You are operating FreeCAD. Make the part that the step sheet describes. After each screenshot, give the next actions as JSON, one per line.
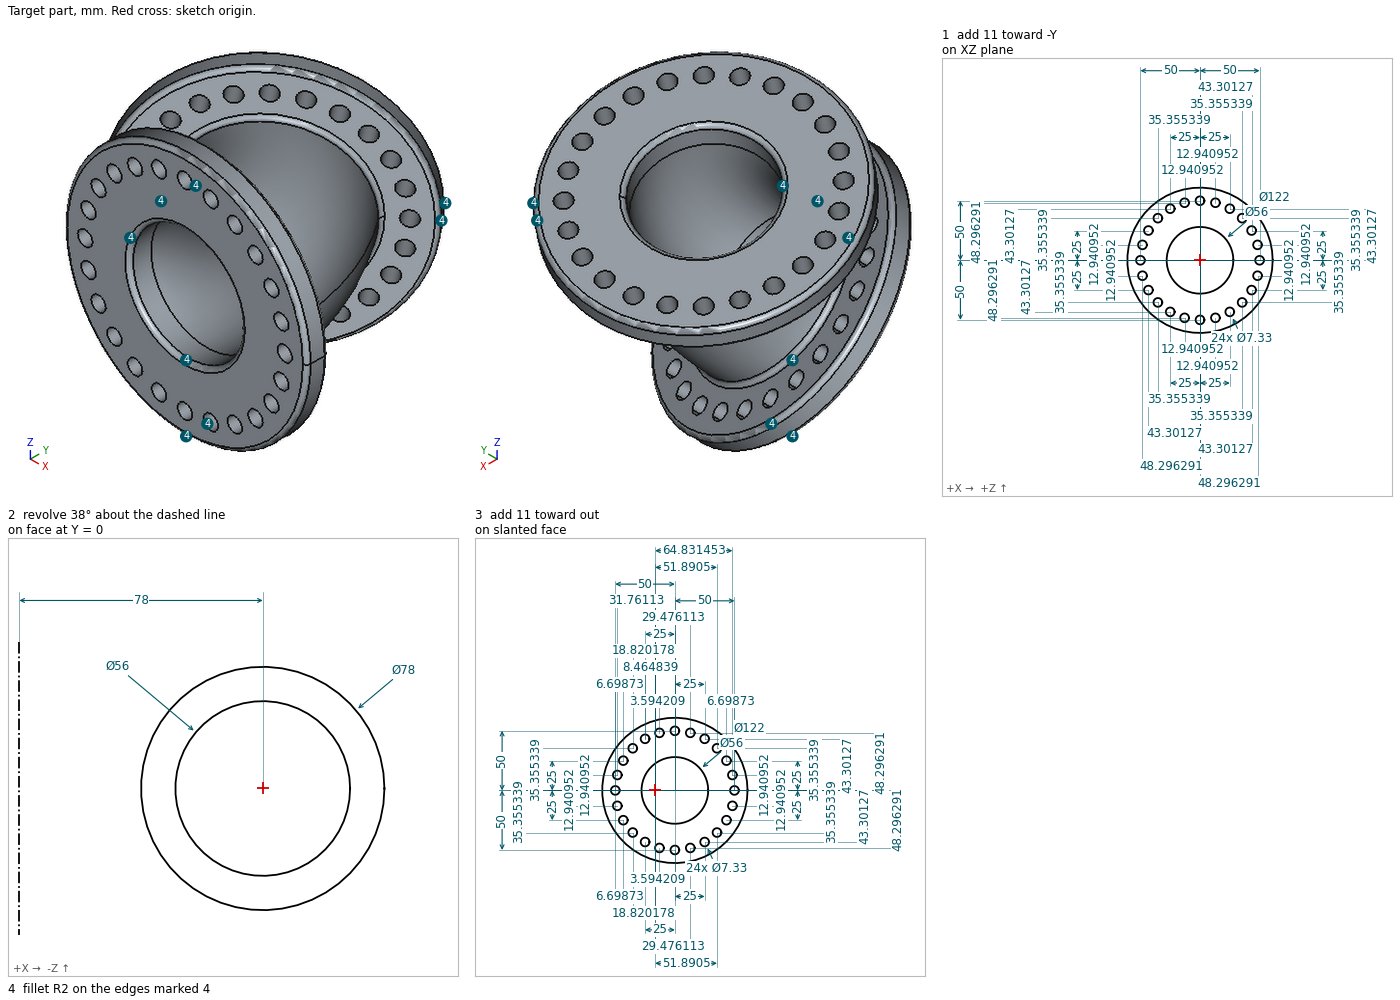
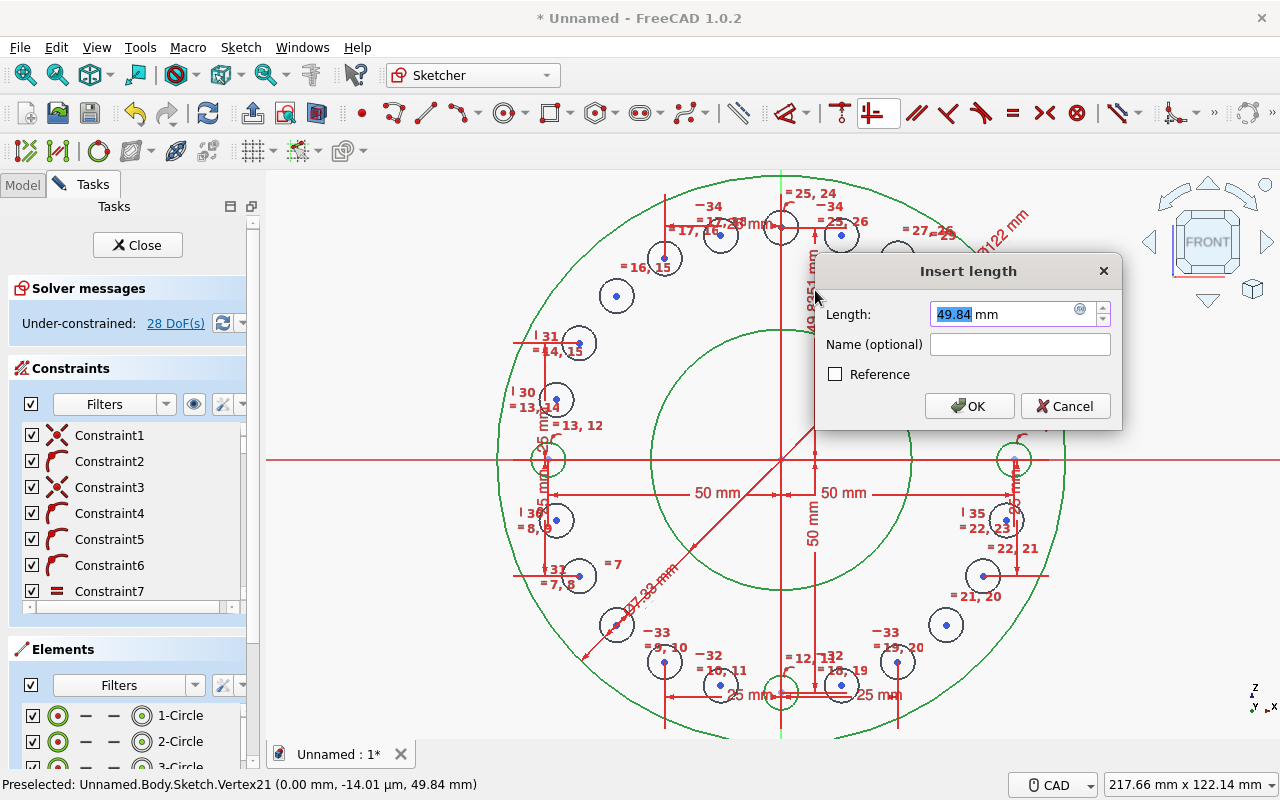
{"action": "type", "text": "50"}
{"action": "key", "text": "Return"}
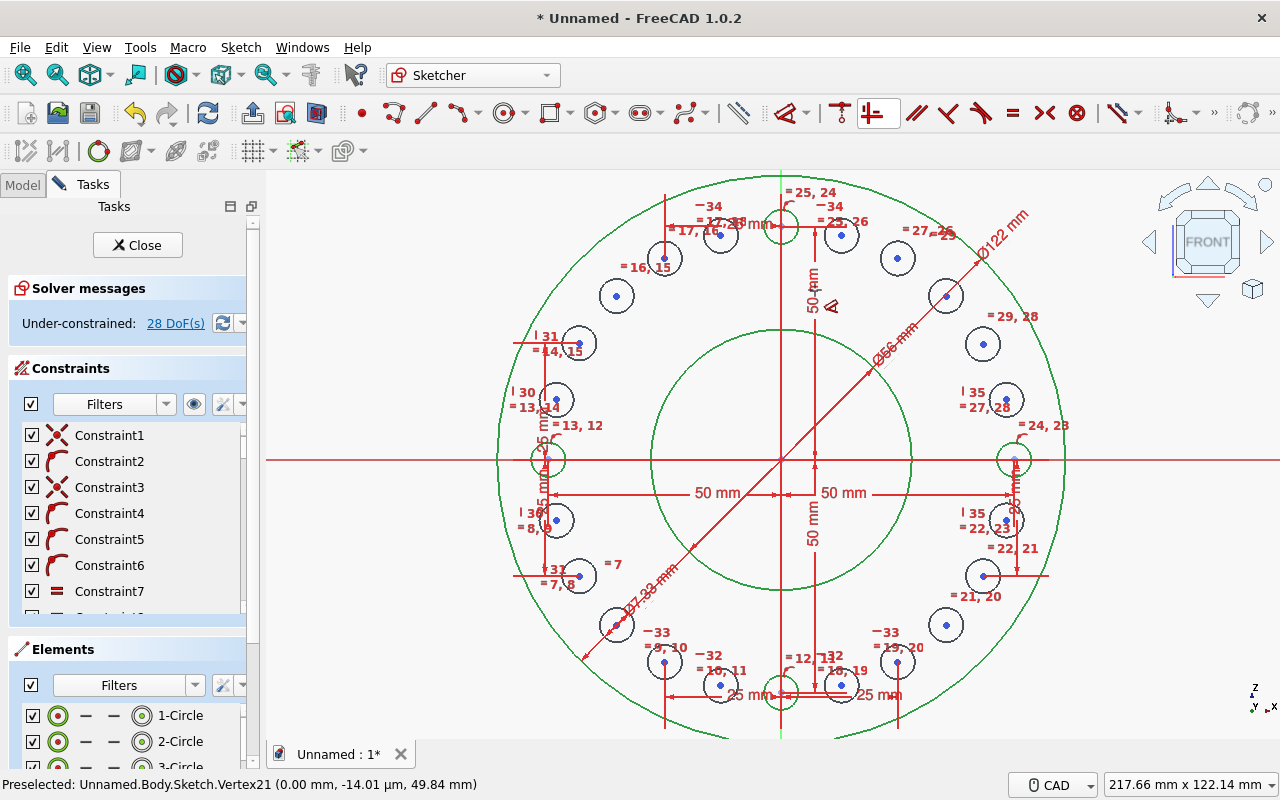
{"action": "left_click", "coordinate": [898, 258]}
{"action": "left_click", "coordinate": [880, 224]}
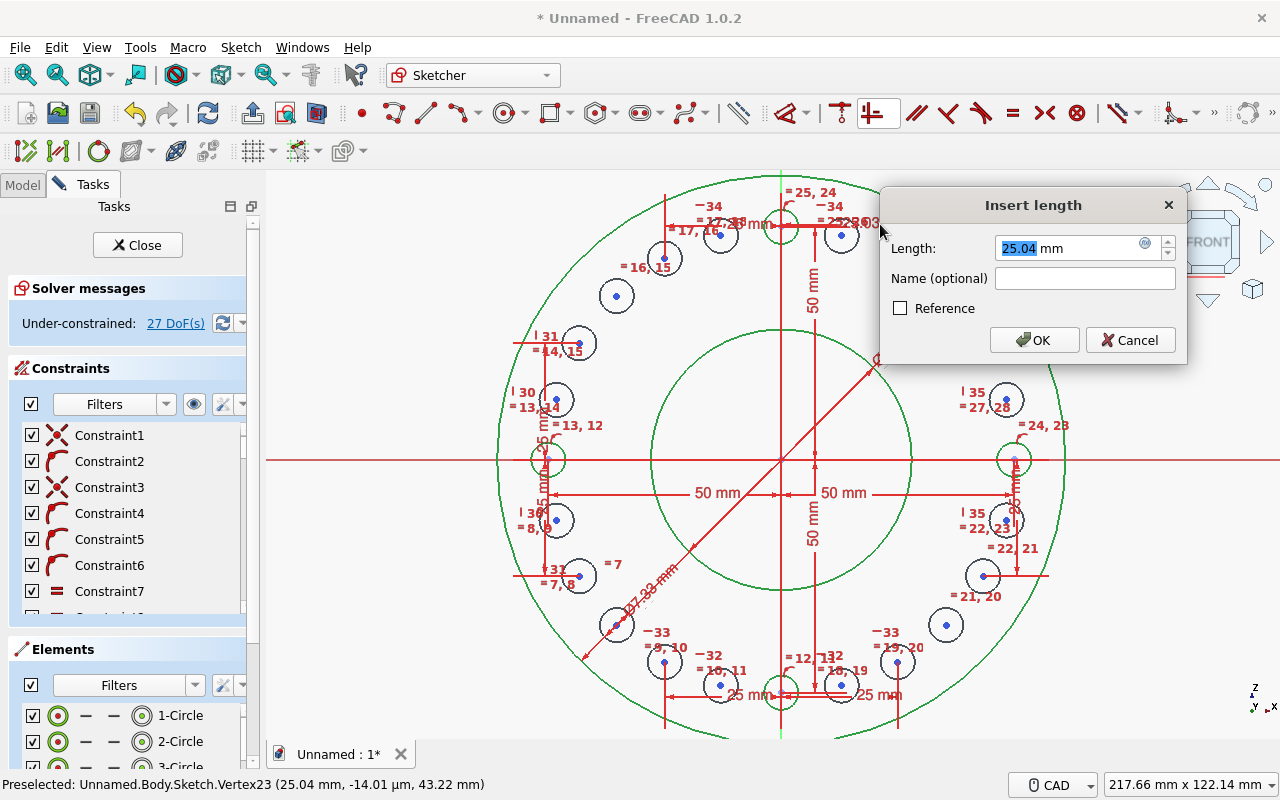
{"action": "type", "text": "25"}
{"action": "key", "text": "Return"}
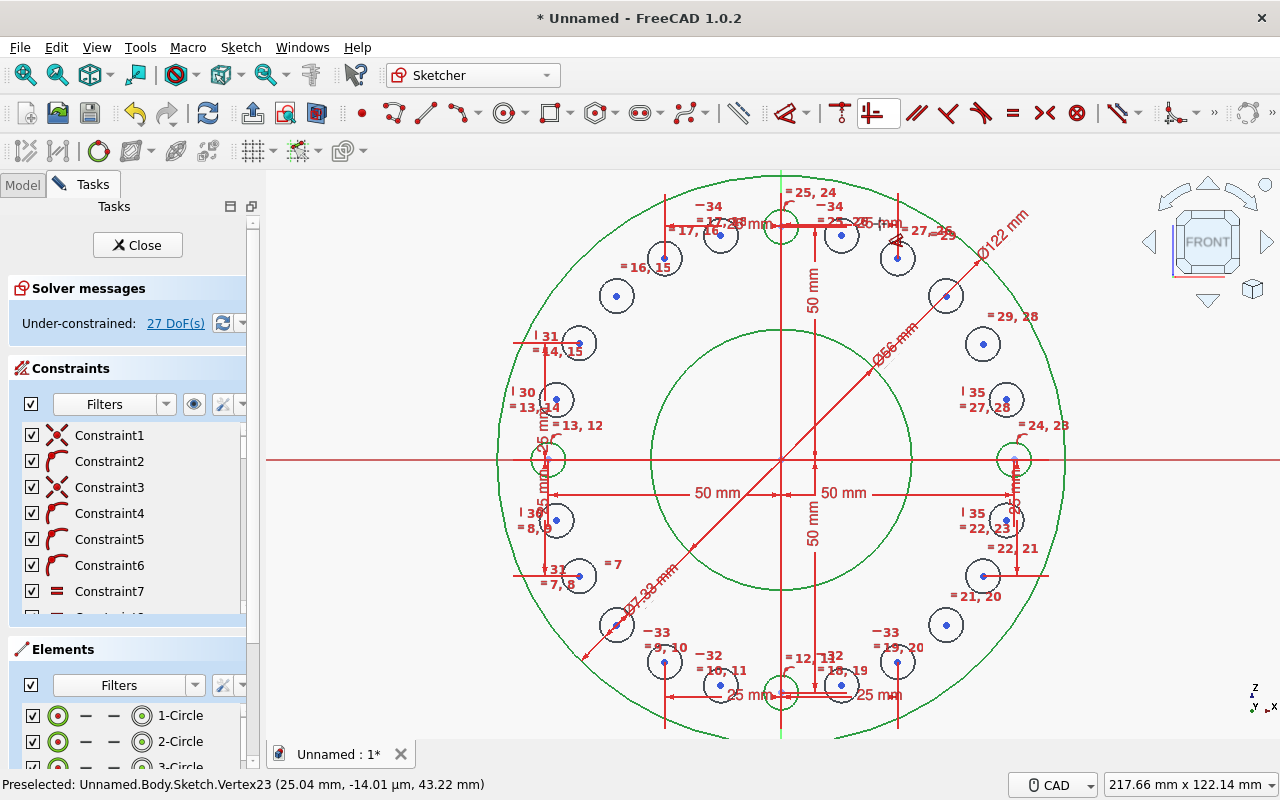
{"action": "left_click", "coordinate": [983, 344]}
{"action": "left_click", "coordinate": [1017, 429]}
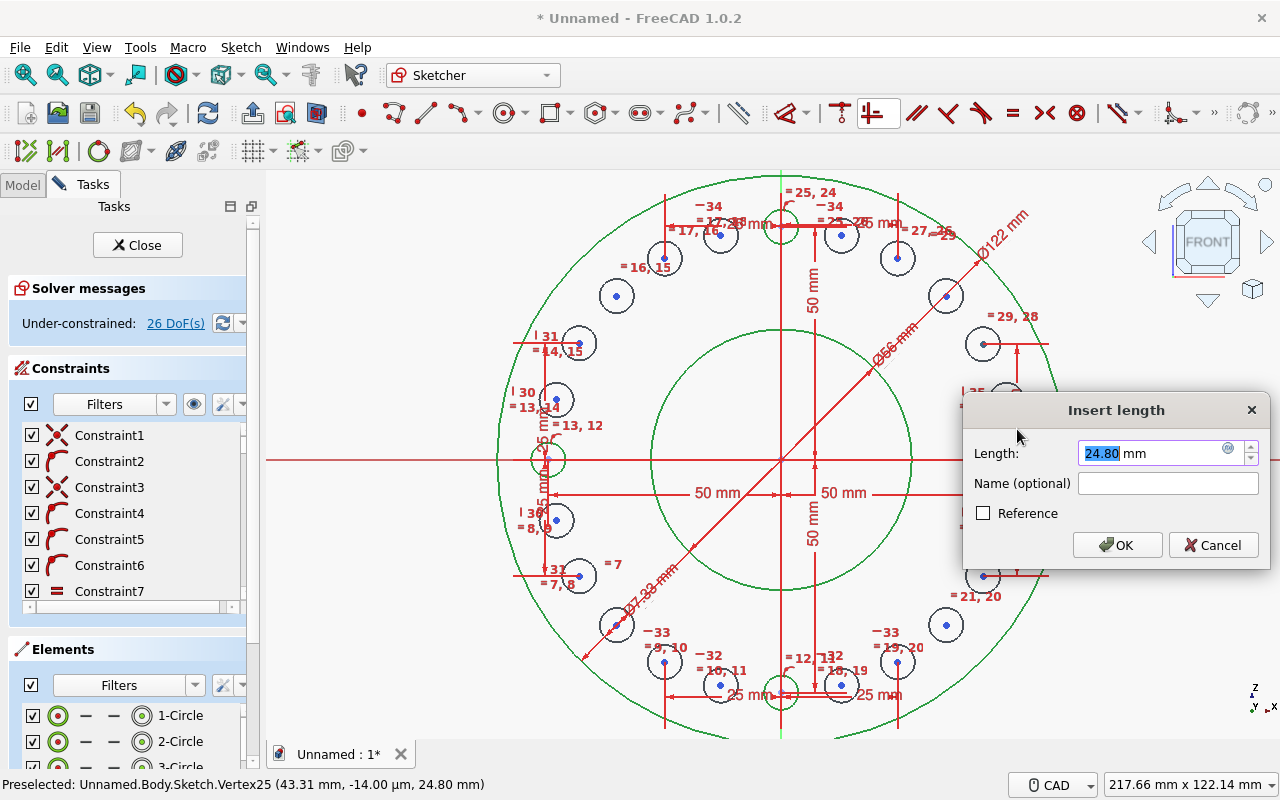
{"action": "type", "text": "25"}
{"action": "key", "text": "Return"}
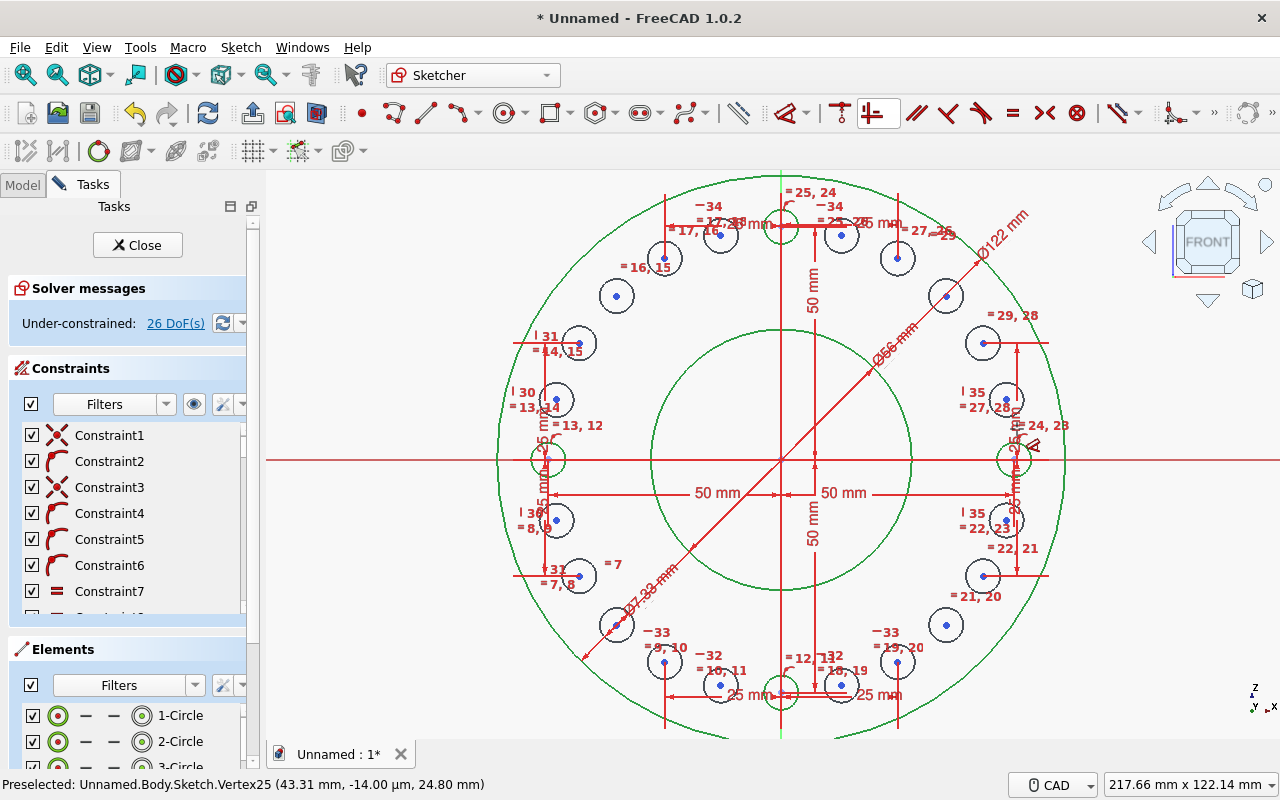
{"action": "left_click", "coordinate": [579, 576]}
{"action": "left_click", "coordinate": [727, 610]}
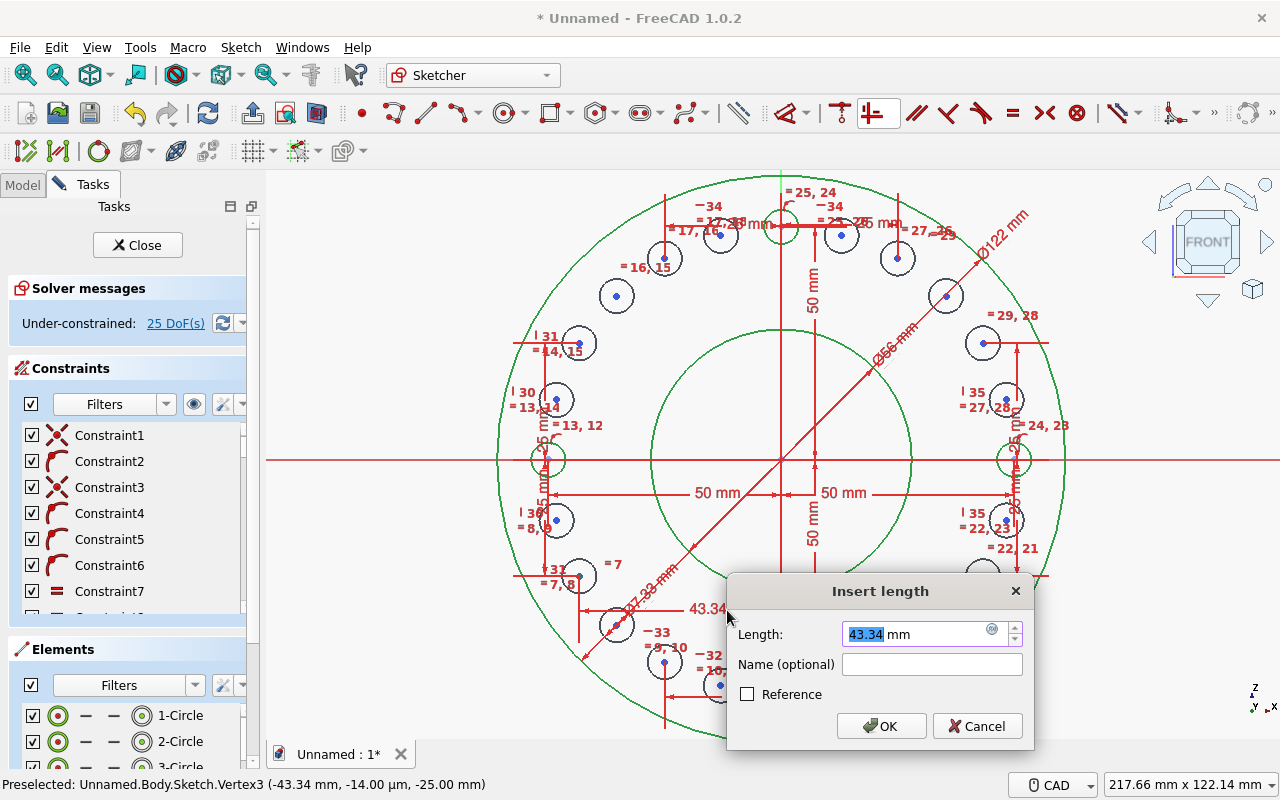
{"action": "type", "text": "43.30127"}
{"action": "key", "text": "Return"}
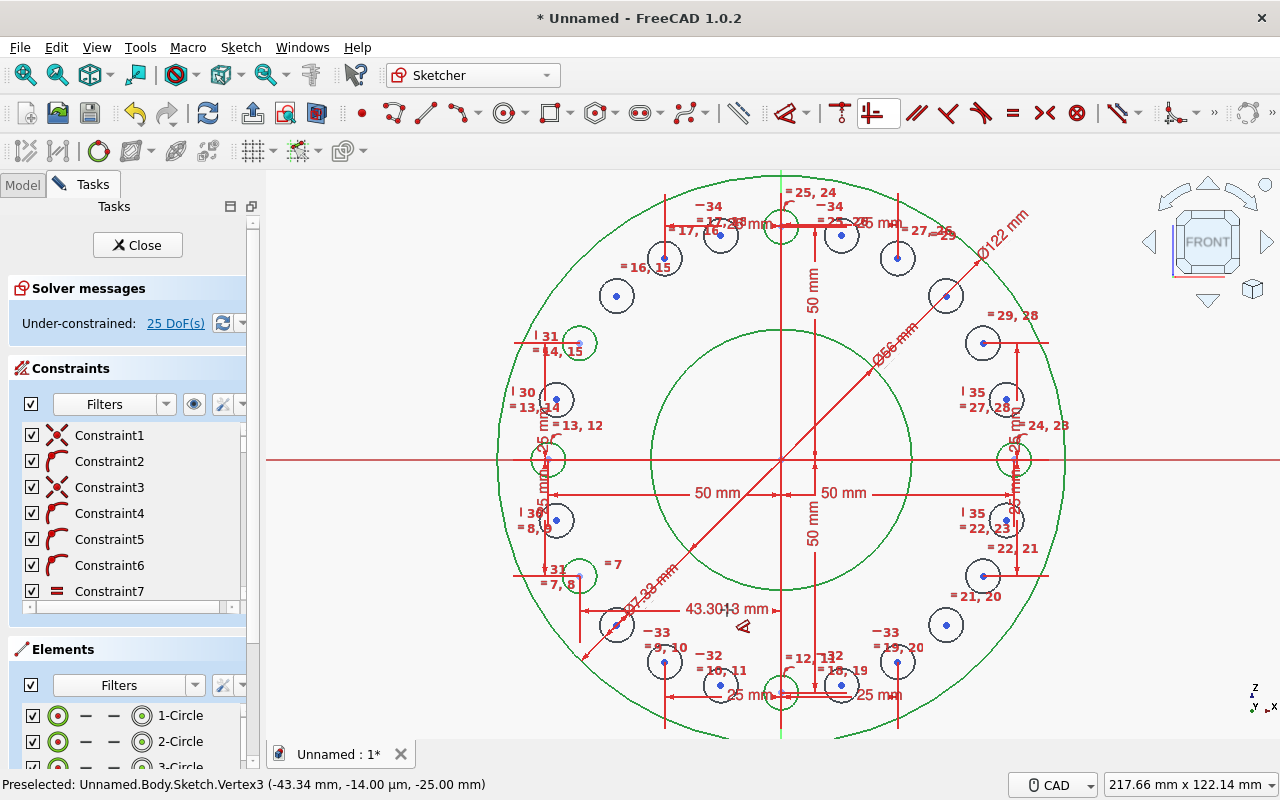
{"action": "left_click", "coordinate": [665, 662]}
{"action": "left_click", "coordinate": [631, 561]}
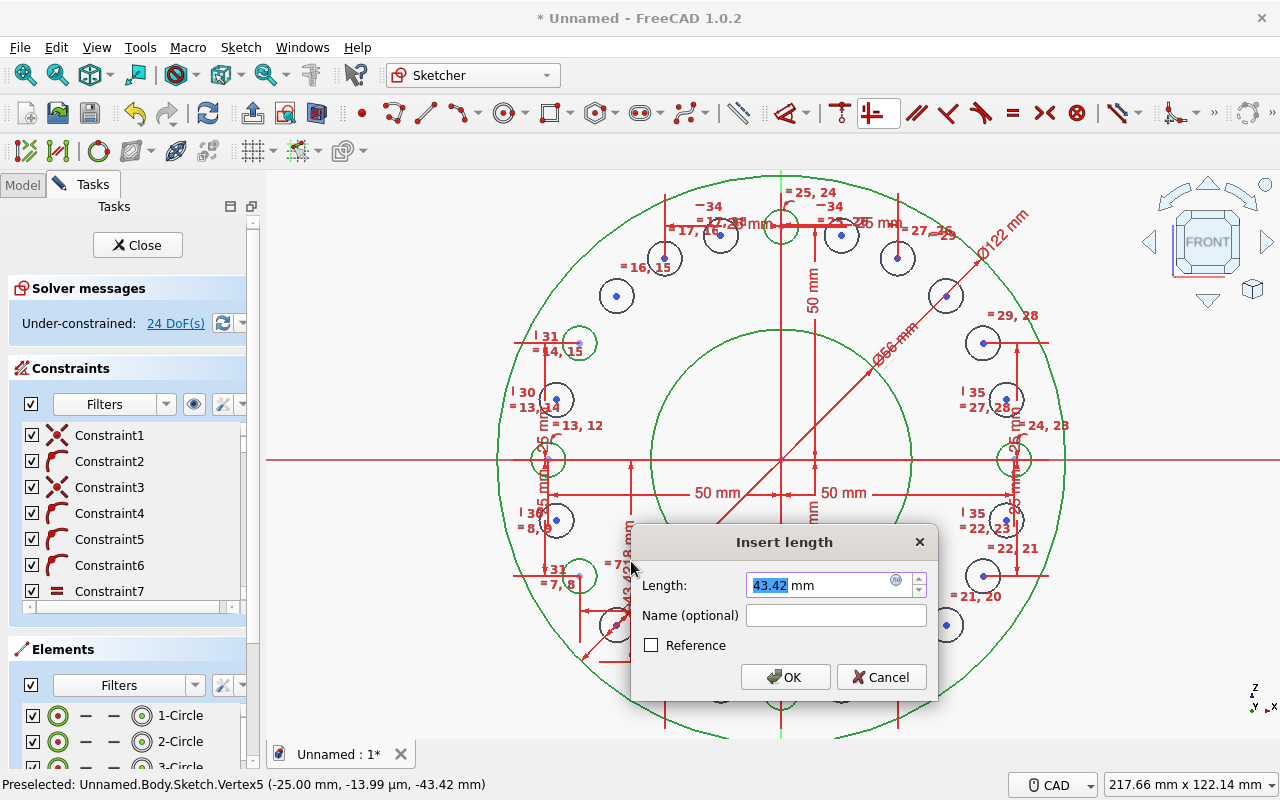
{"action": "type", "text": "43.30127"}
{"action": "key", "text": "Return"}